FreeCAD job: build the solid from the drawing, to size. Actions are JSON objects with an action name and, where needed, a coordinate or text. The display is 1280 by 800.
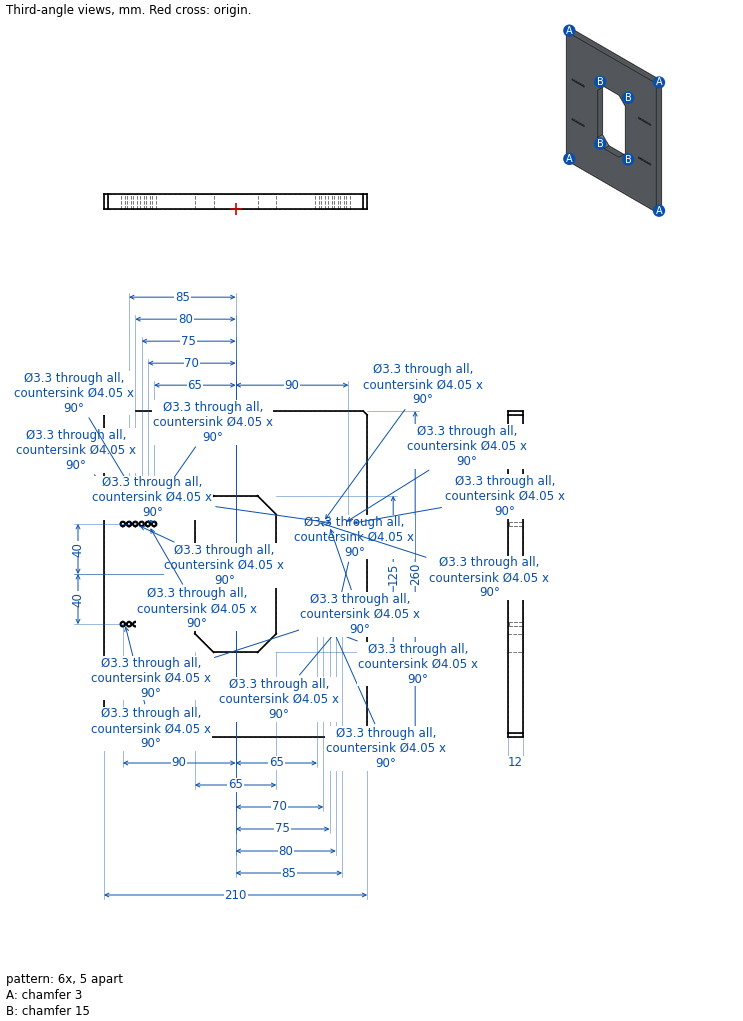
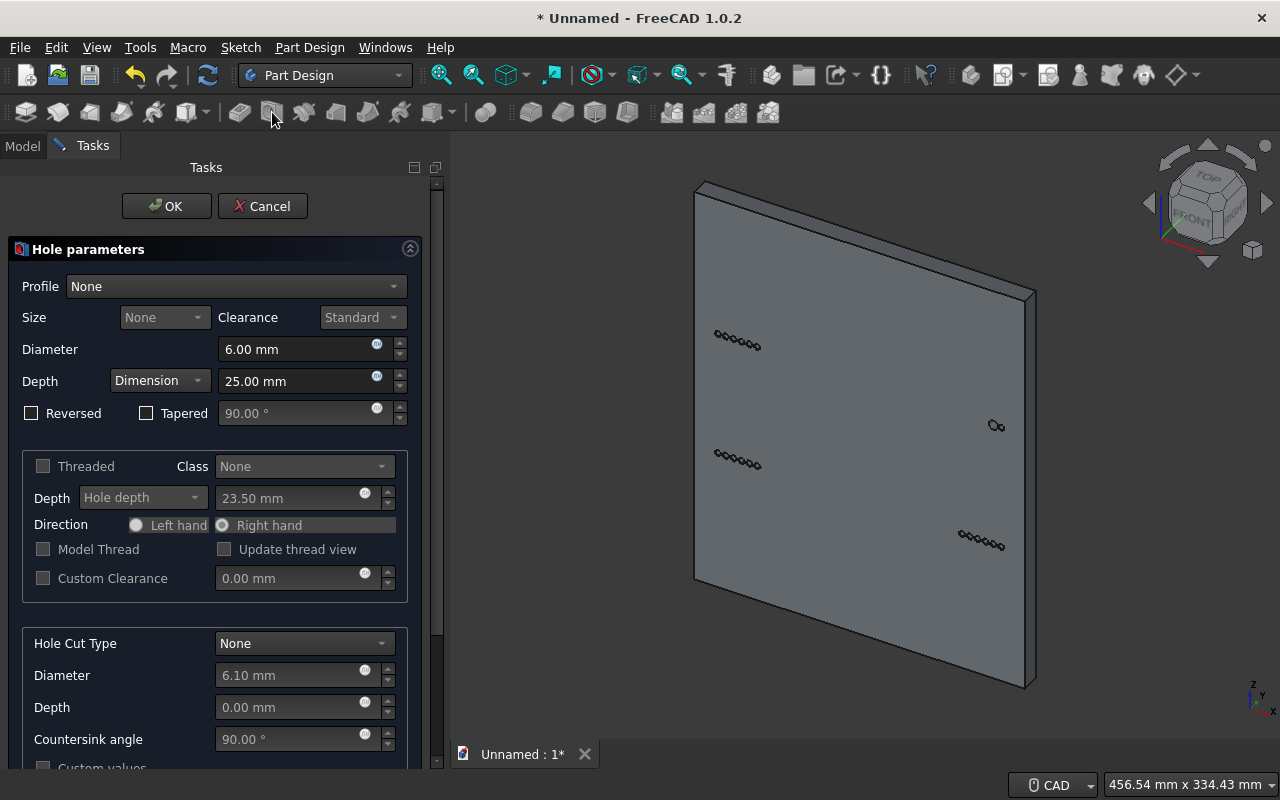
{"action": "triple_click", "coordinate": [305, 349]}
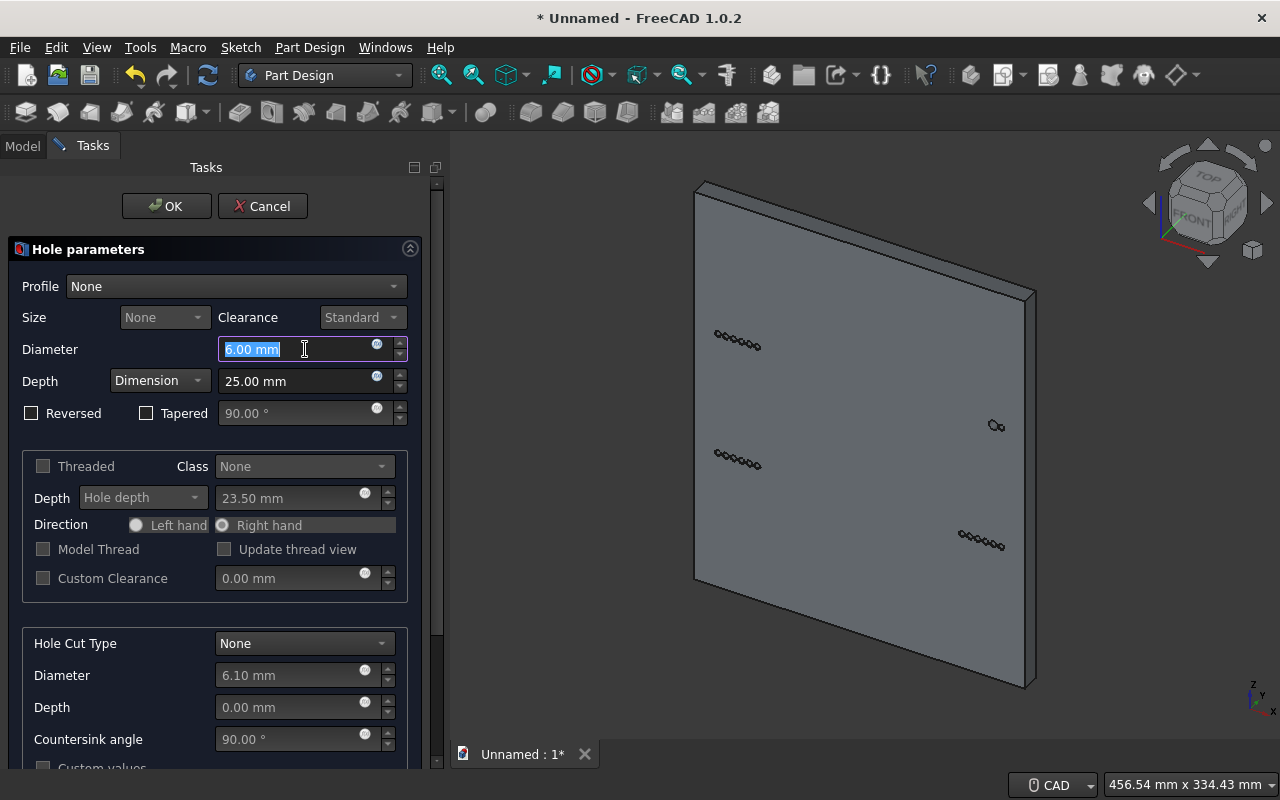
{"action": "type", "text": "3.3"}
{"action": "key", "text": "Tab"}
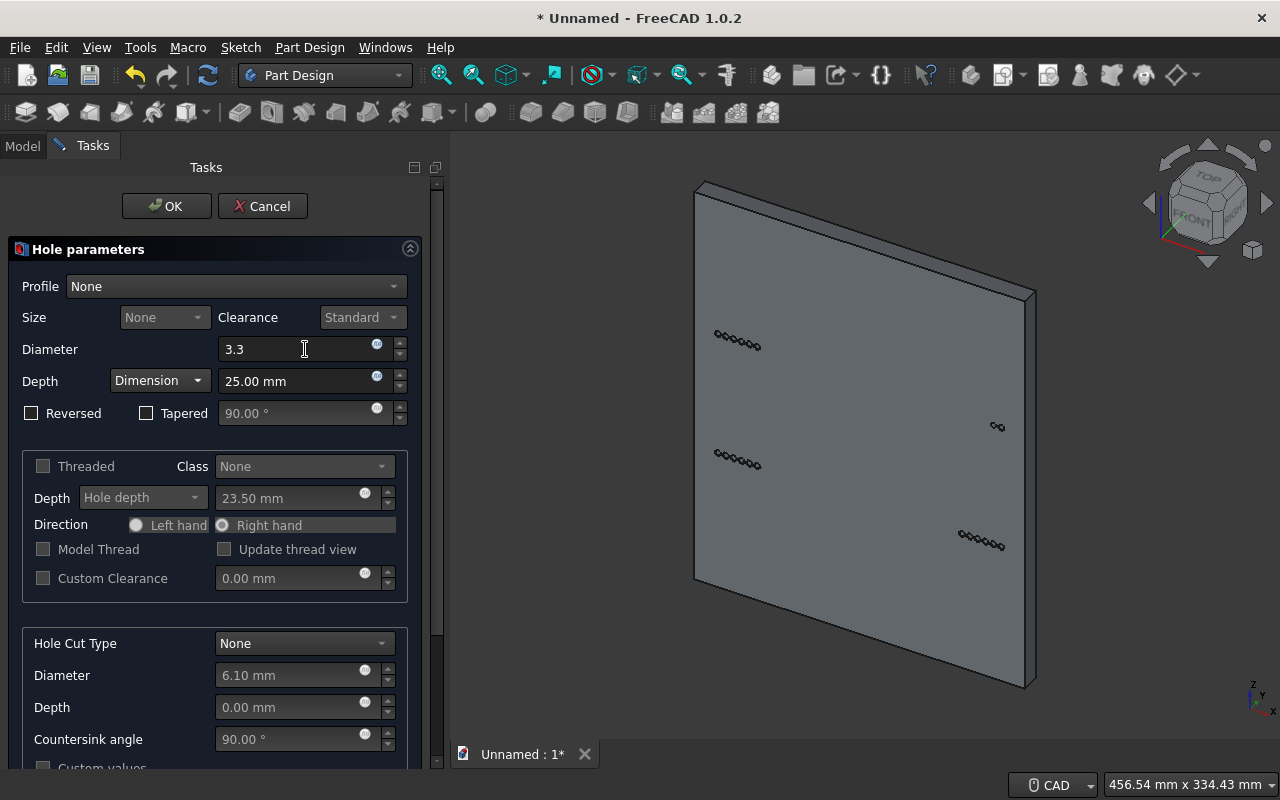
{"action": "left_click", "coordinate": [161, 380]}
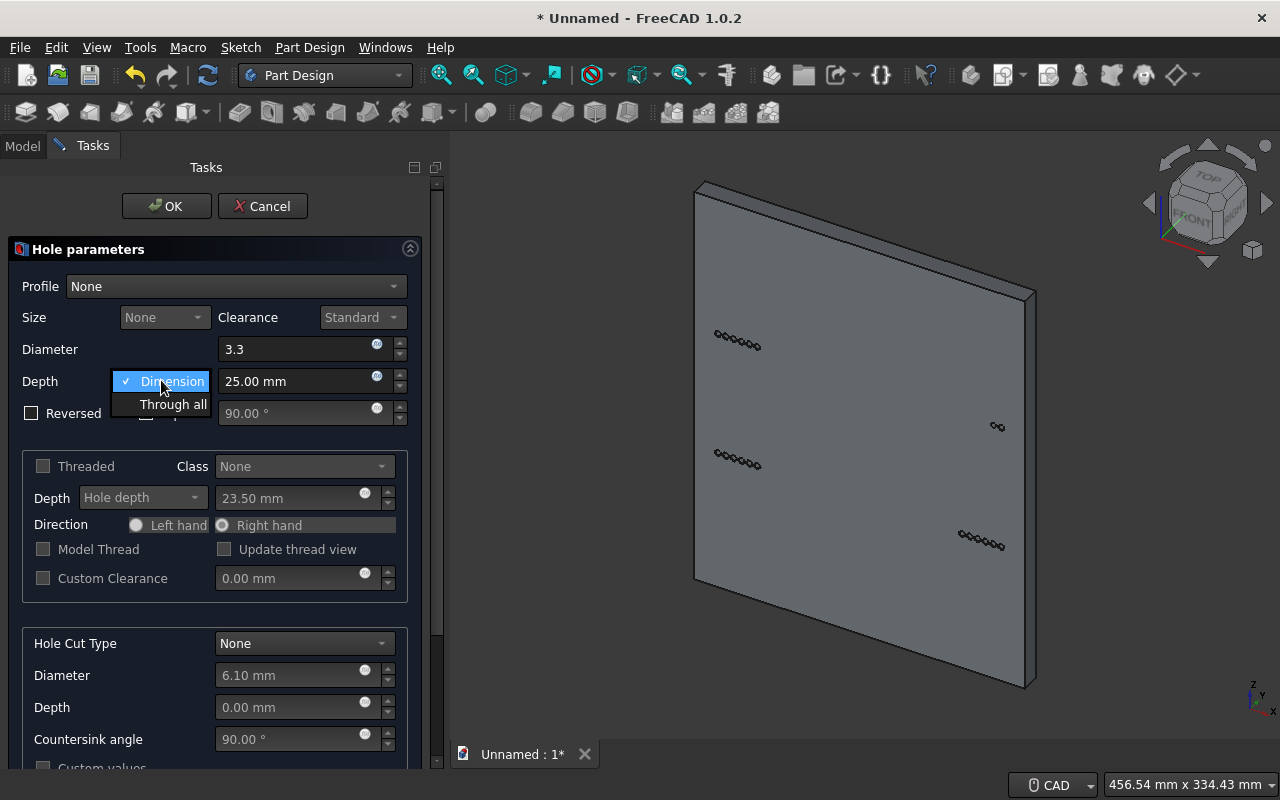
{"action": "left_click", "coordinate": [160, 404]}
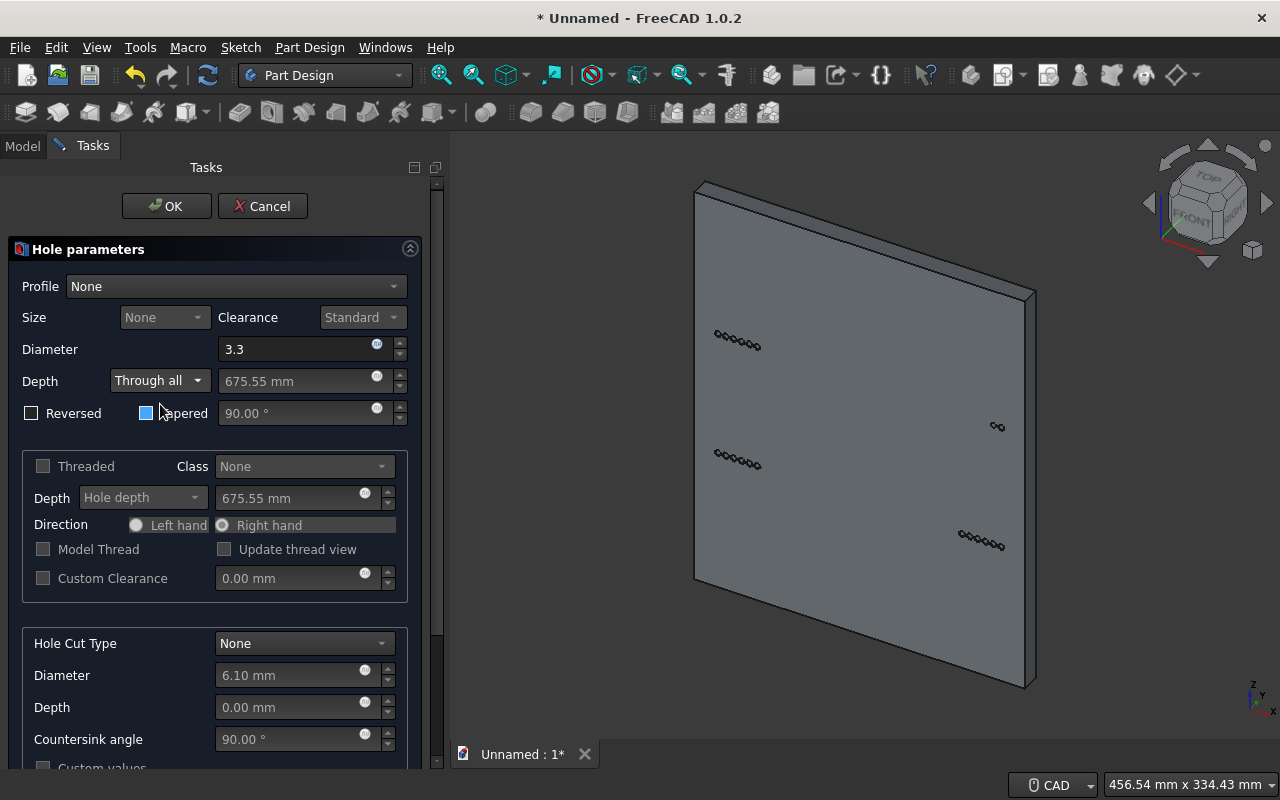
{"action": "left_click", "coordinate": [306, 644]}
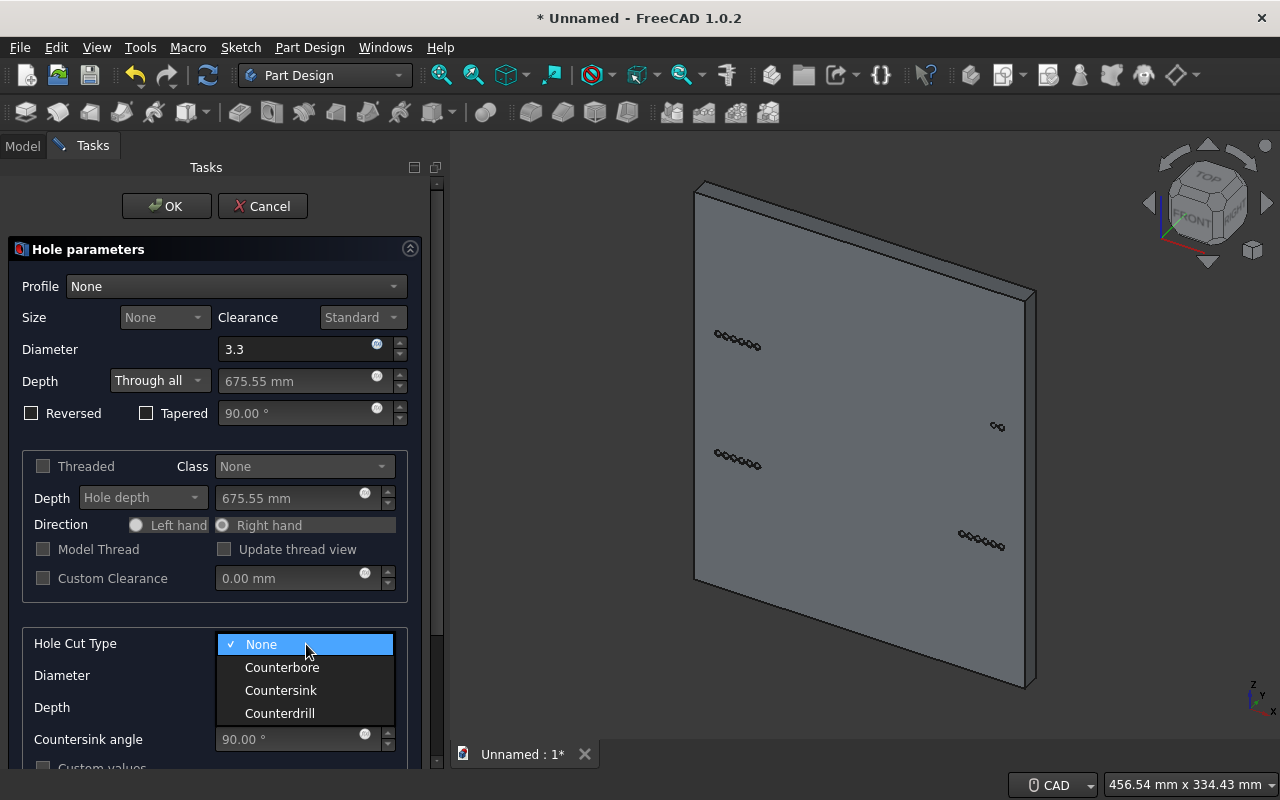
{"action": "left_click", "coordinate": [304, 690]}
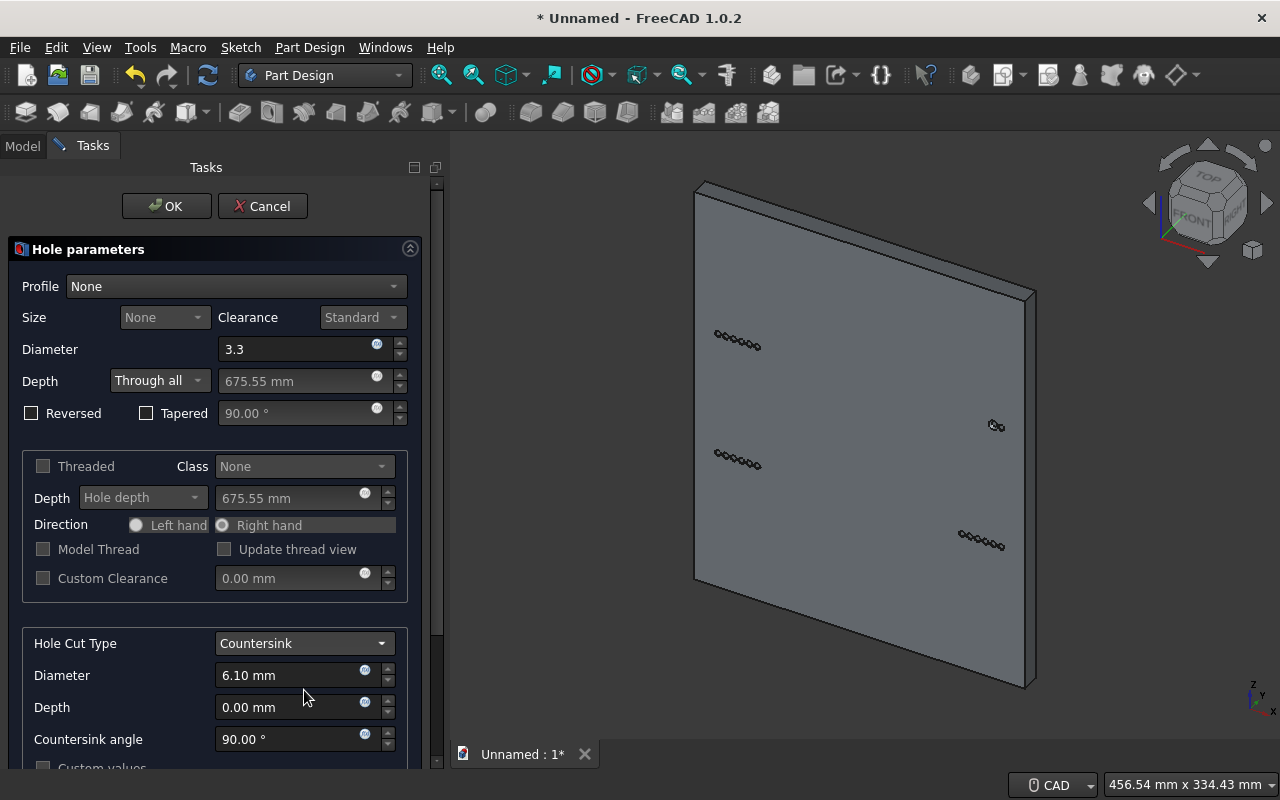
{"action": "triple_click", "coordinate": [298, 675]}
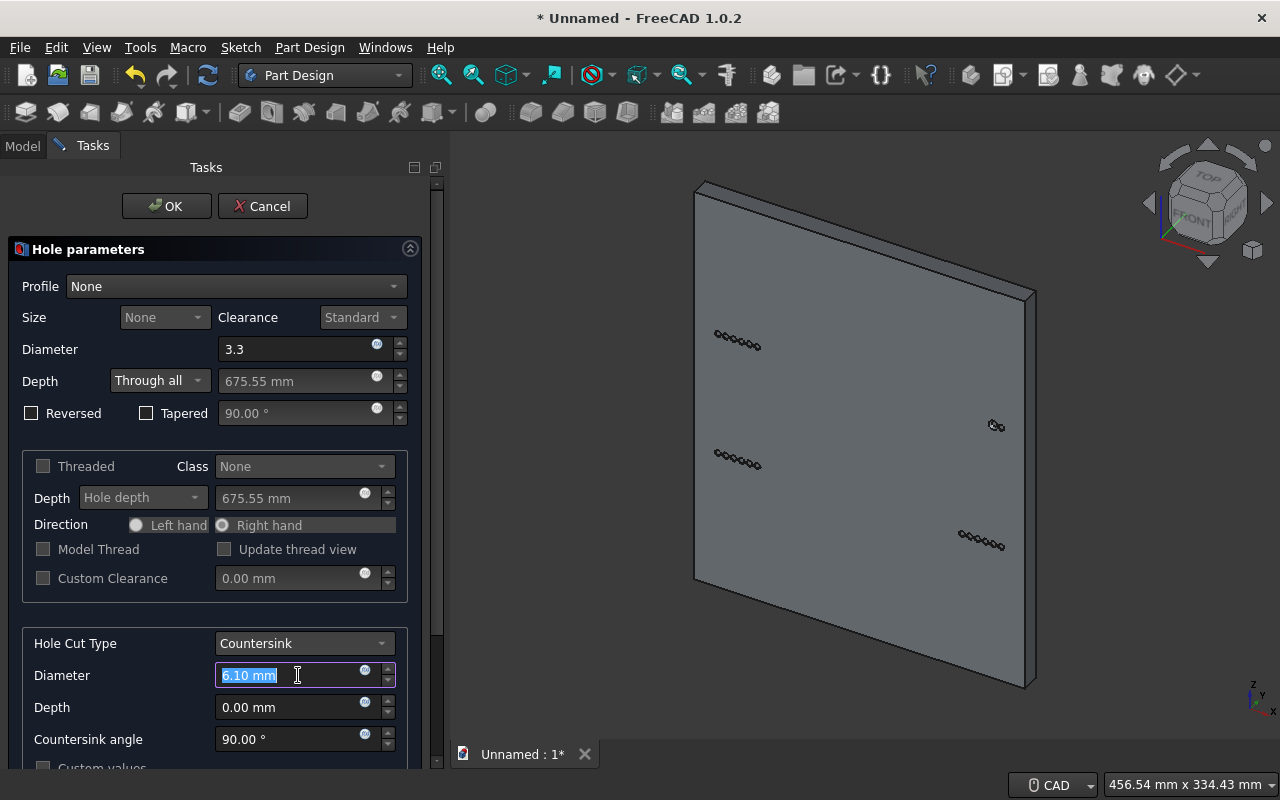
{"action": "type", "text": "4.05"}
{"action": "key", "text": "Tab"}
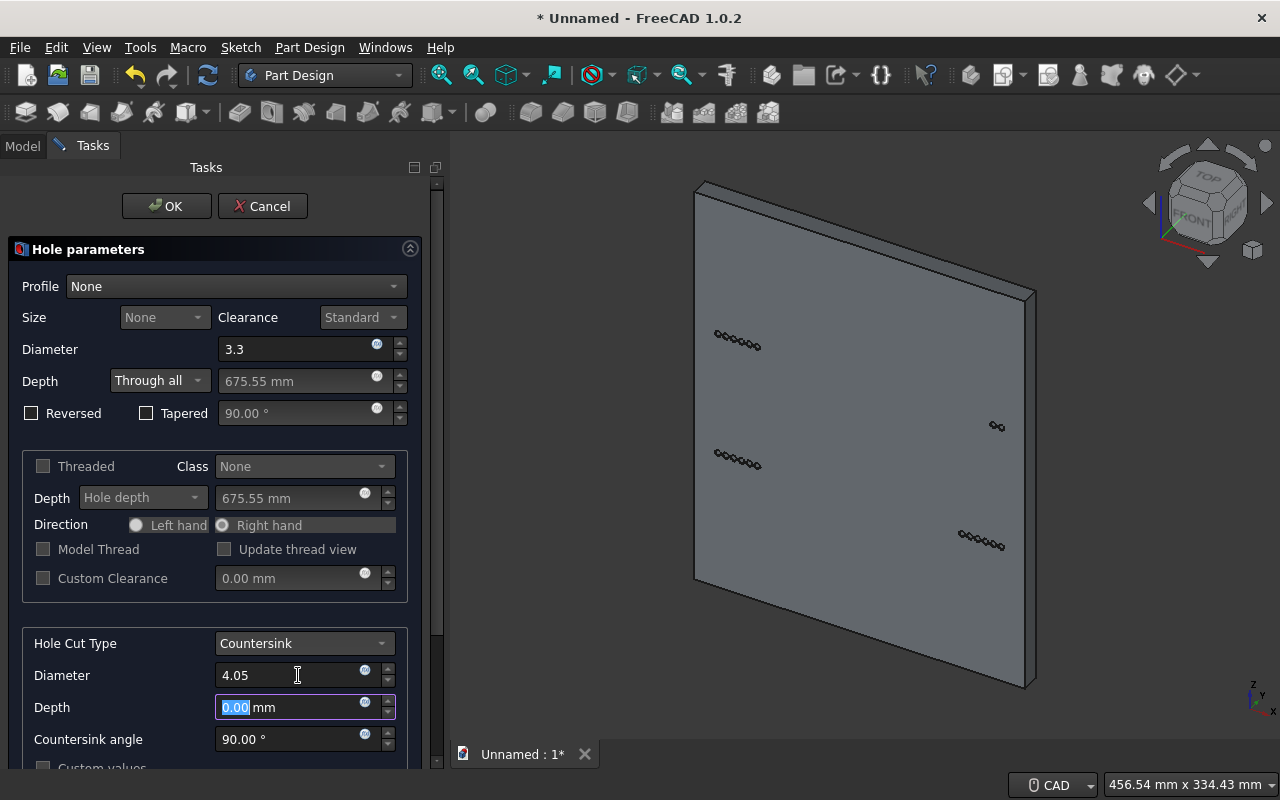
{"action": "left_click", "coordinate": [167, 206]}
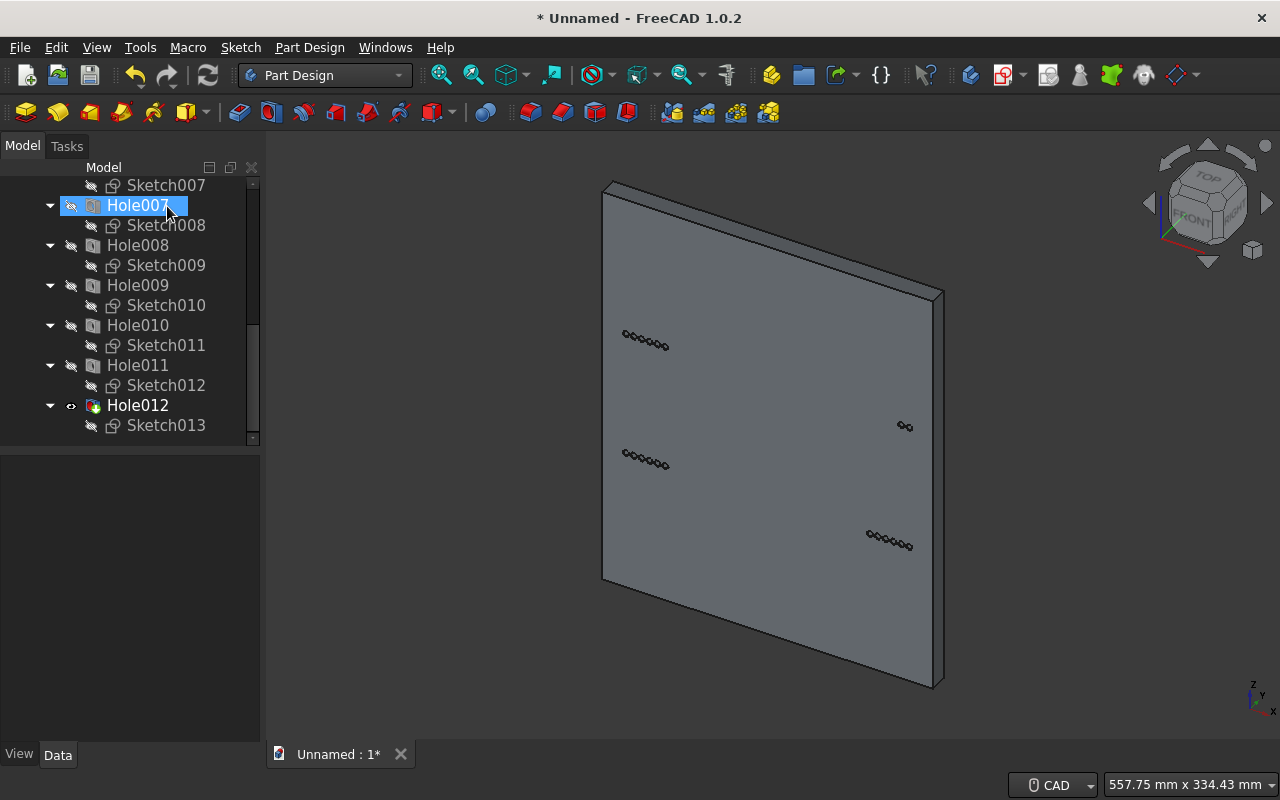
{"action": "left_click", "coordinate": [768, 439]}